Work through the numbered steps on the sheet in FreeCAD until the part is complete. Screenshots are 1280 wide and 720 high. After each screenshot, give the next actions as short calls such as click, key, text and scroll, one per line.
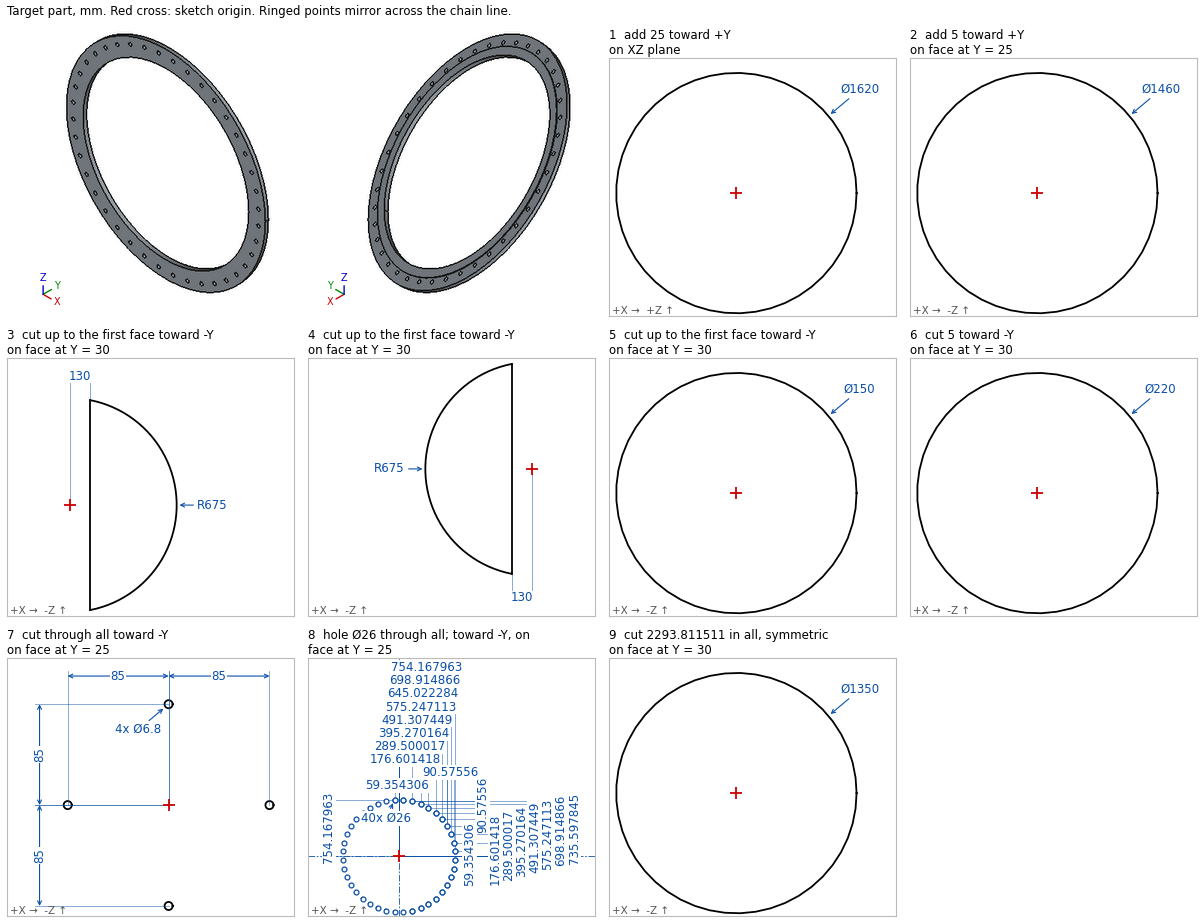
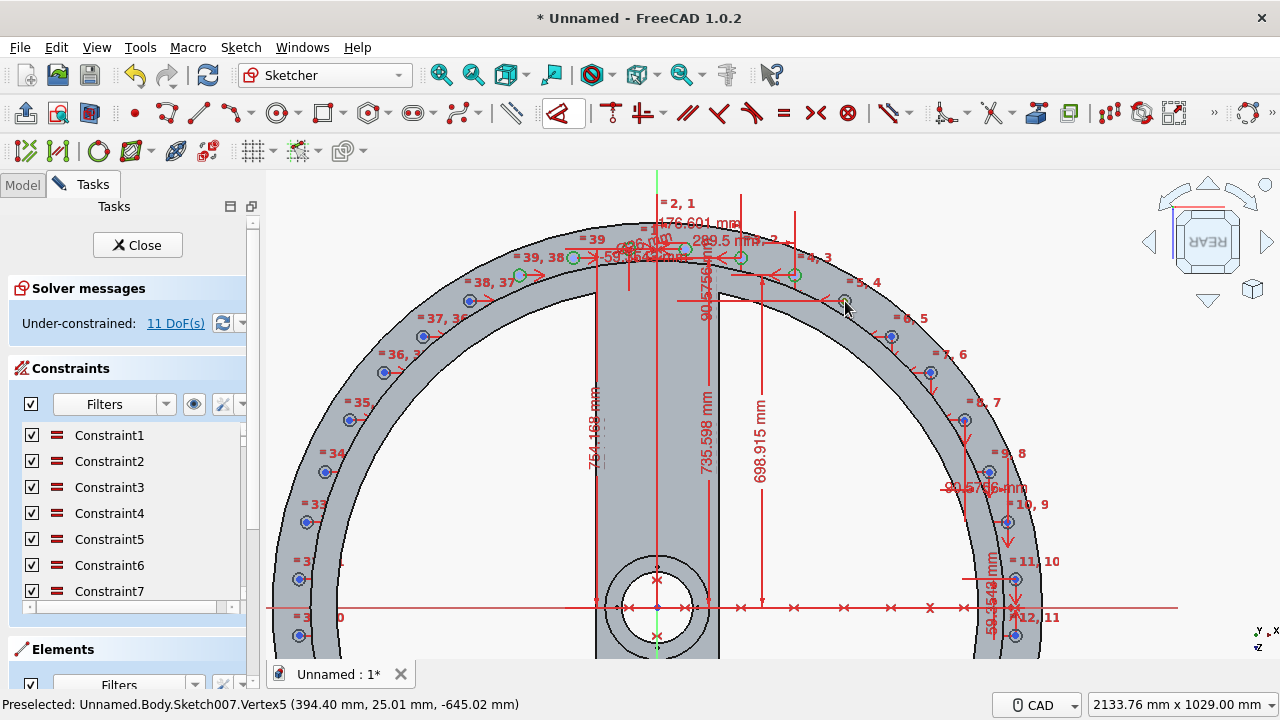
key(l)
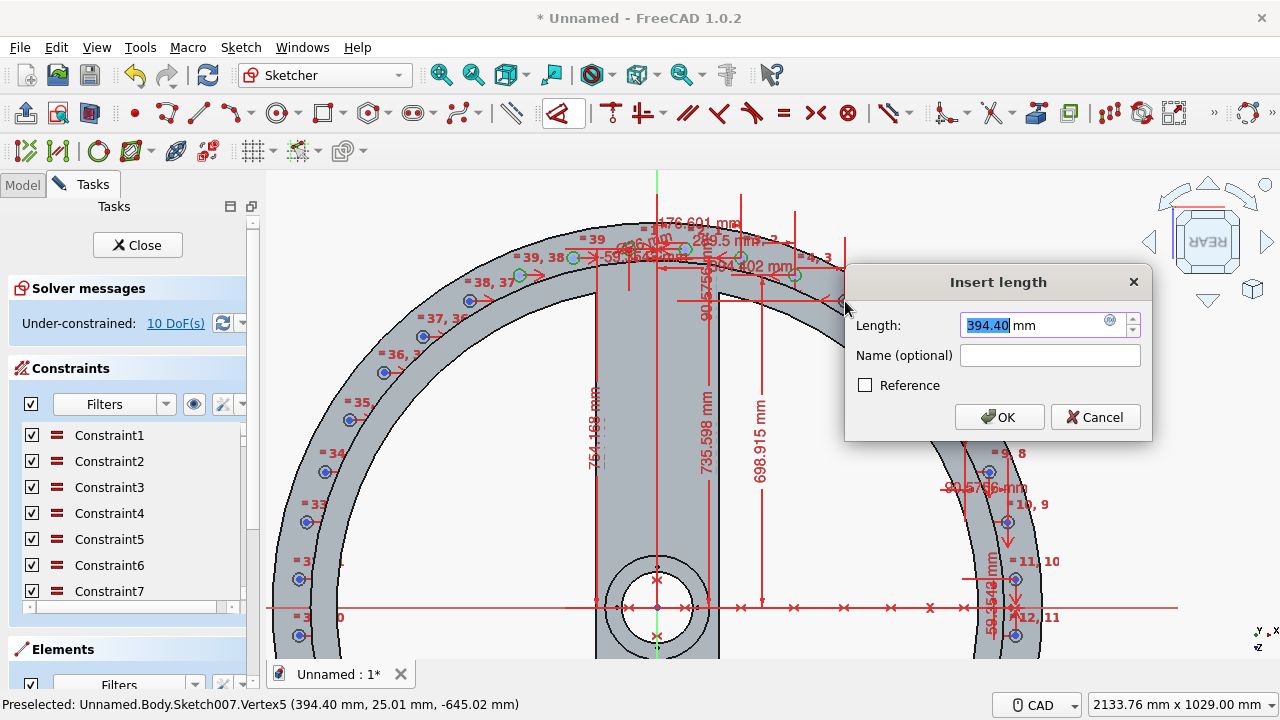
text(395.270164)
key(Return)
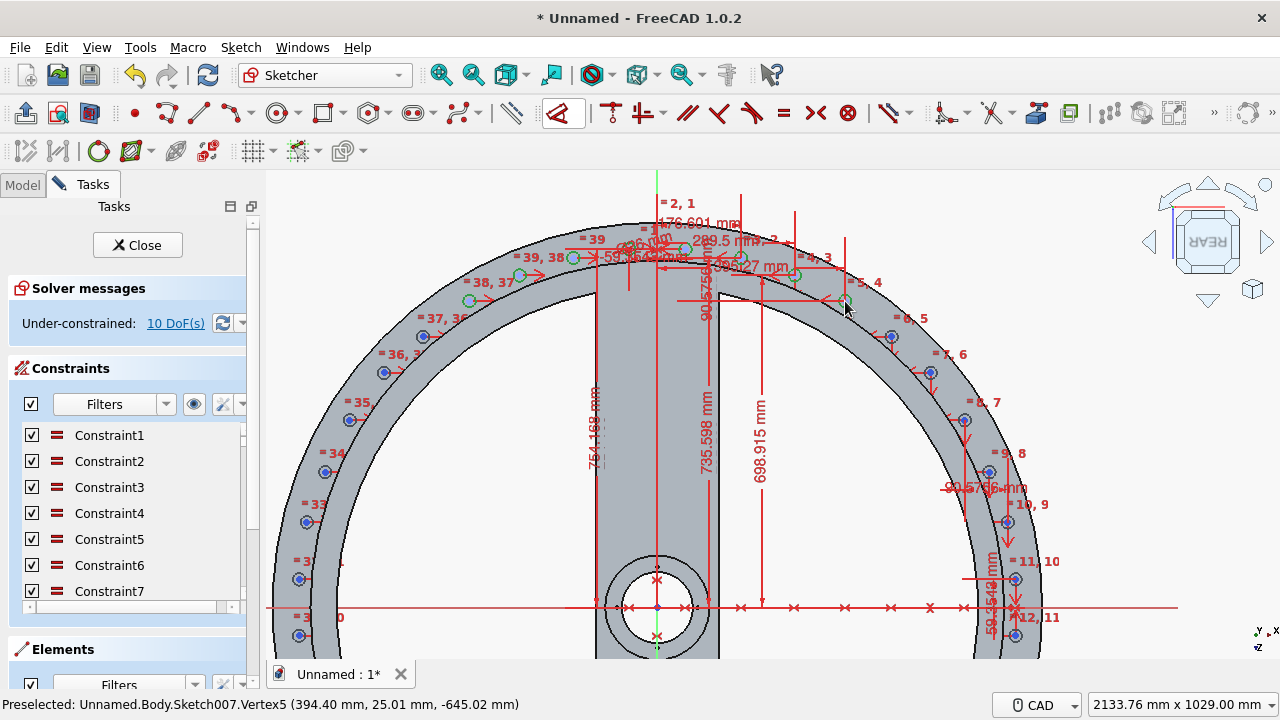
click(892, 337)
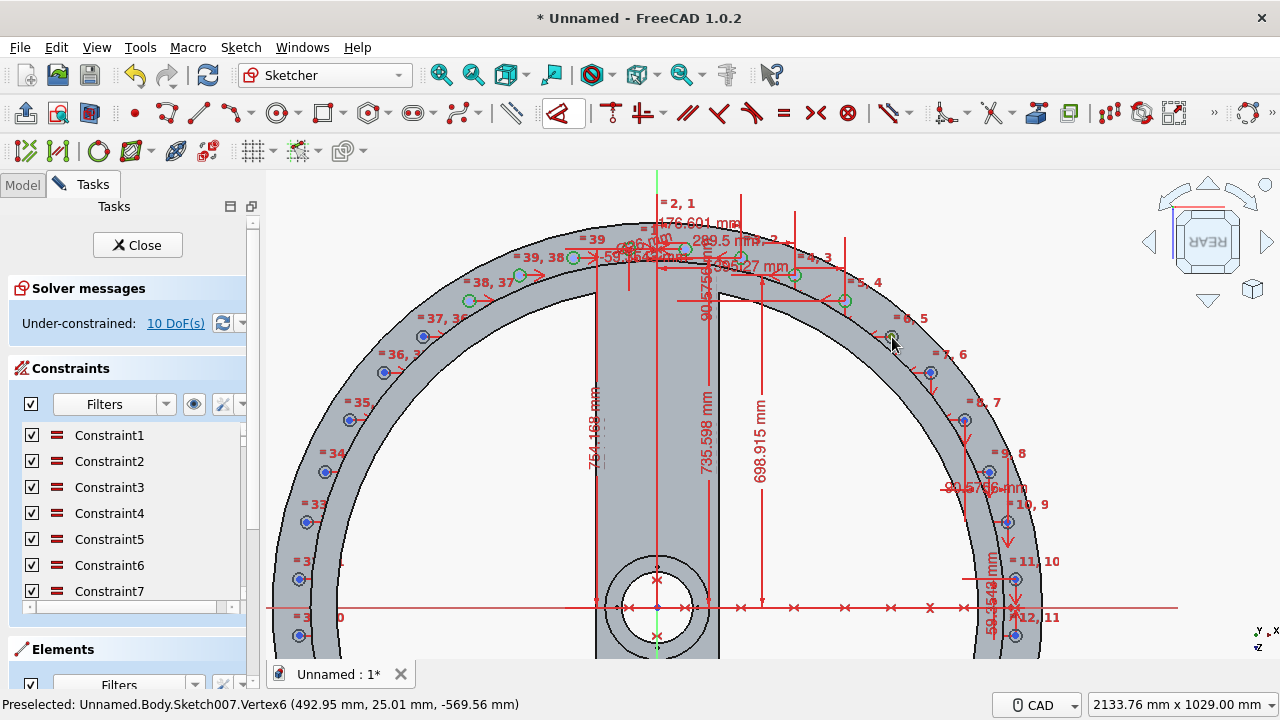
click(580, 114)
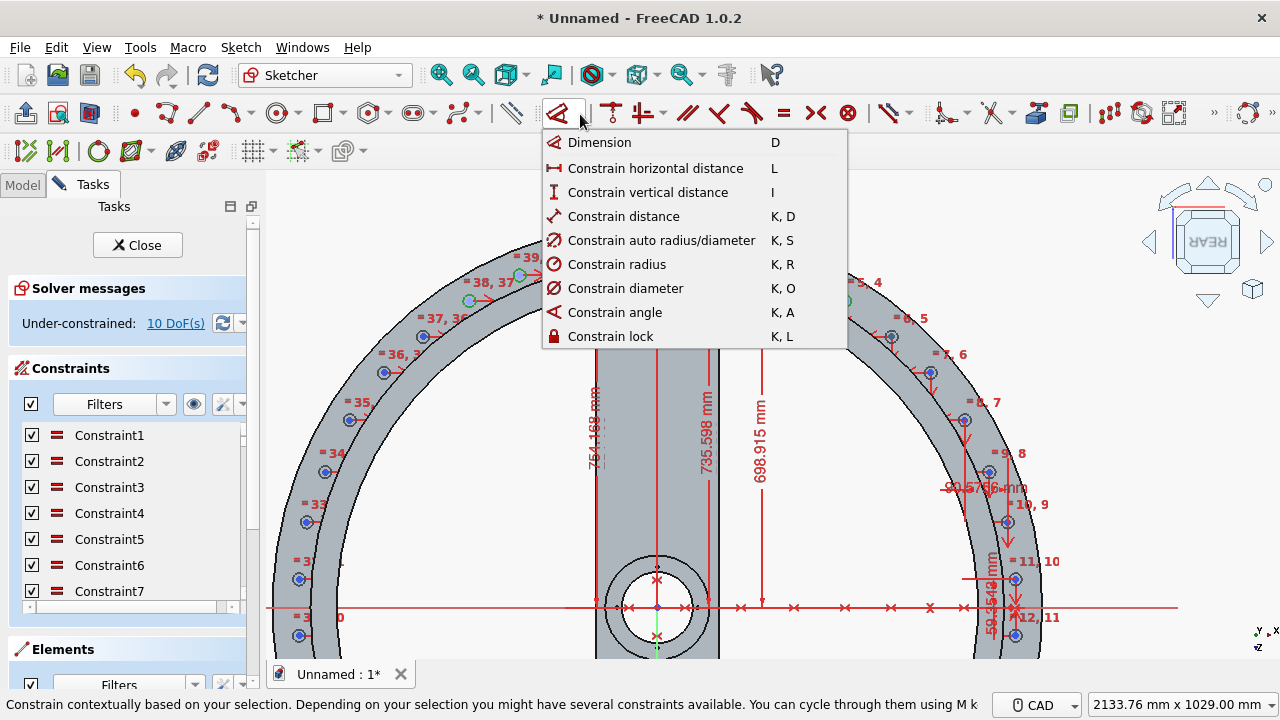
click(695, 168)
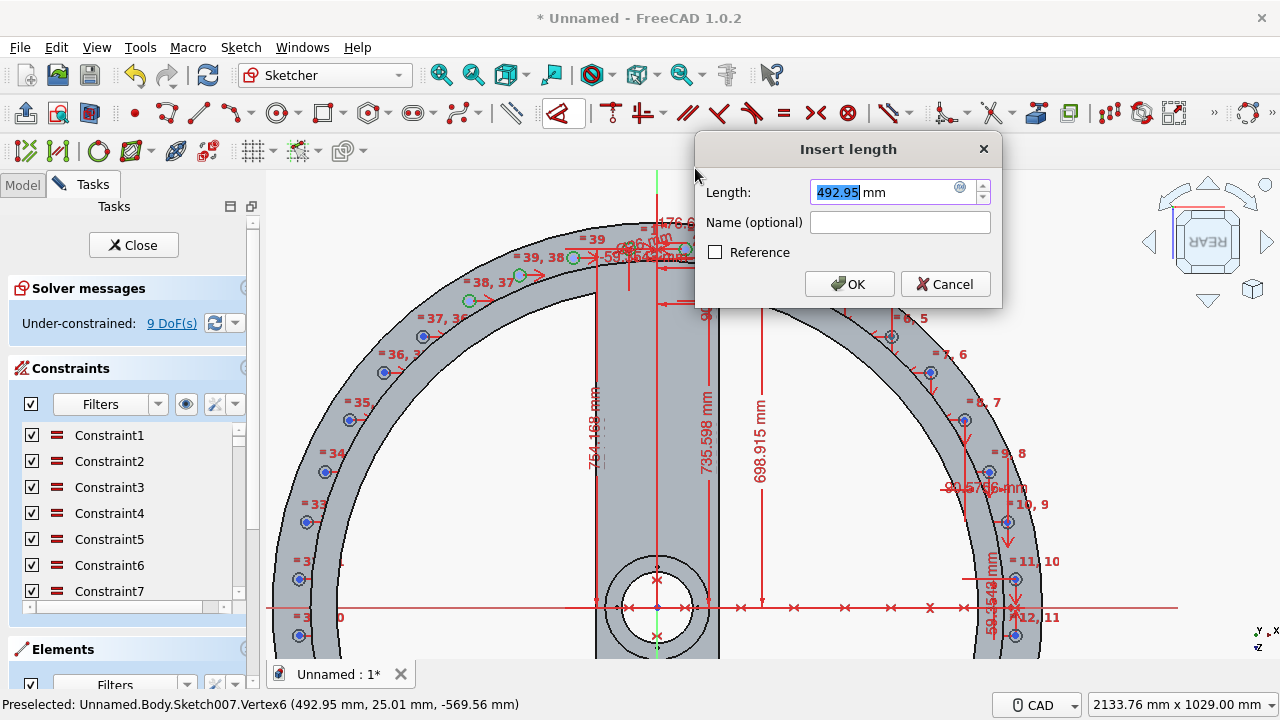
text(491.307449)
key(Return)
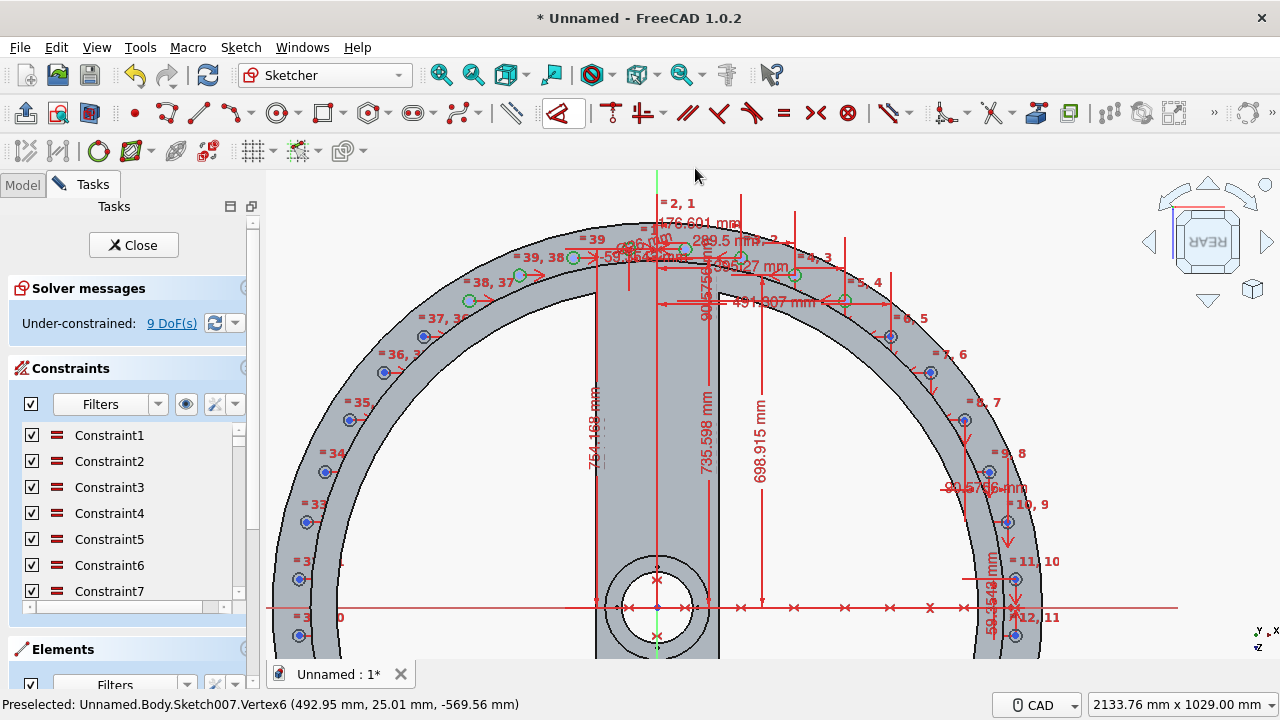
click(891, 337)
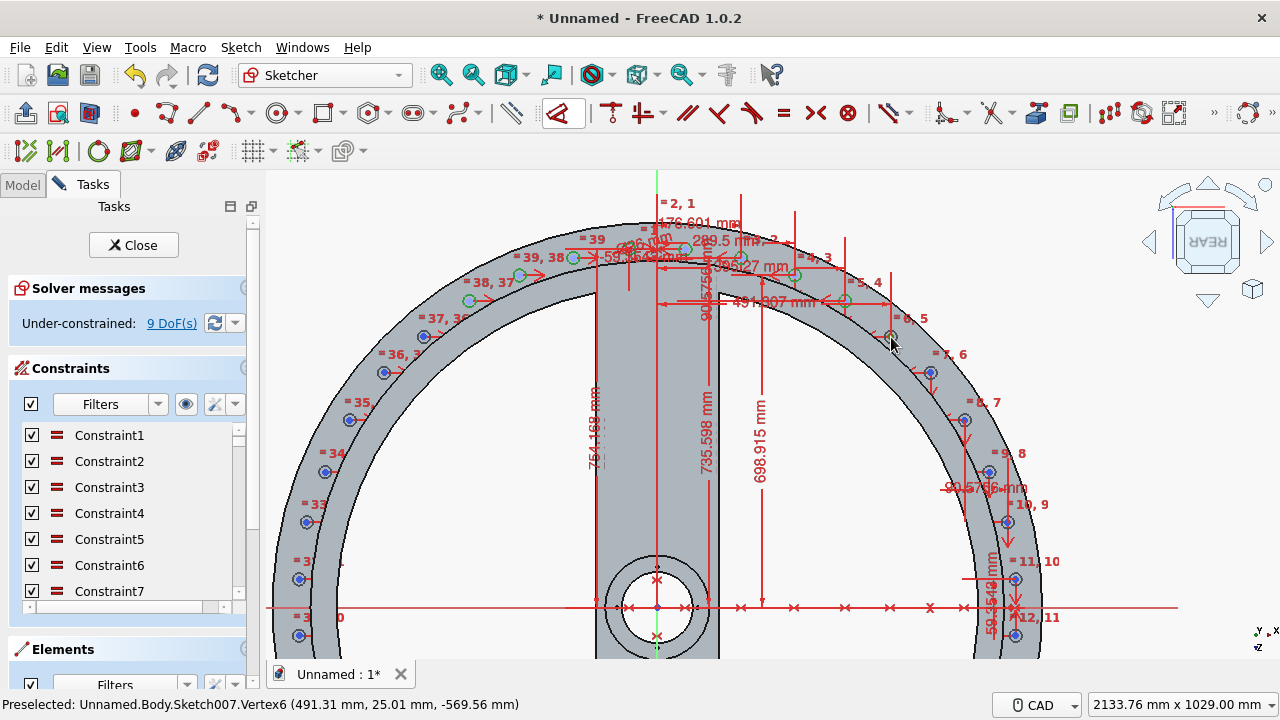
key(i)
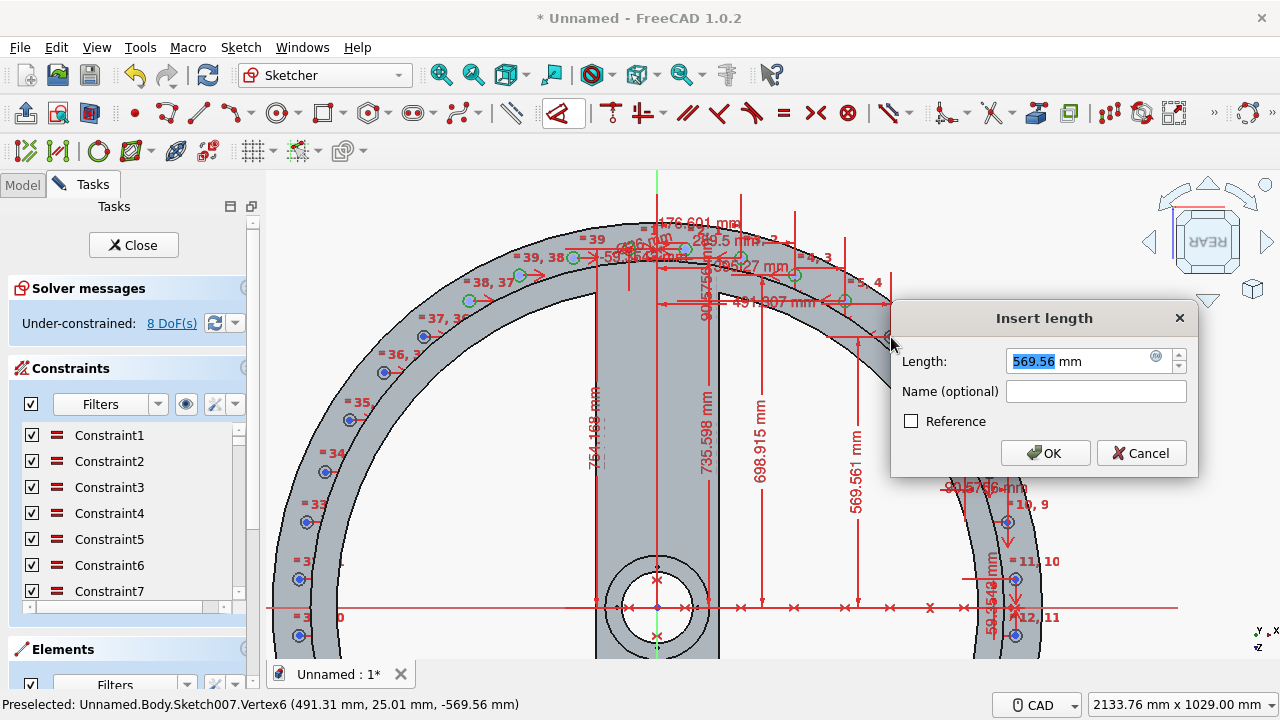
text(575.247113)
key(Return)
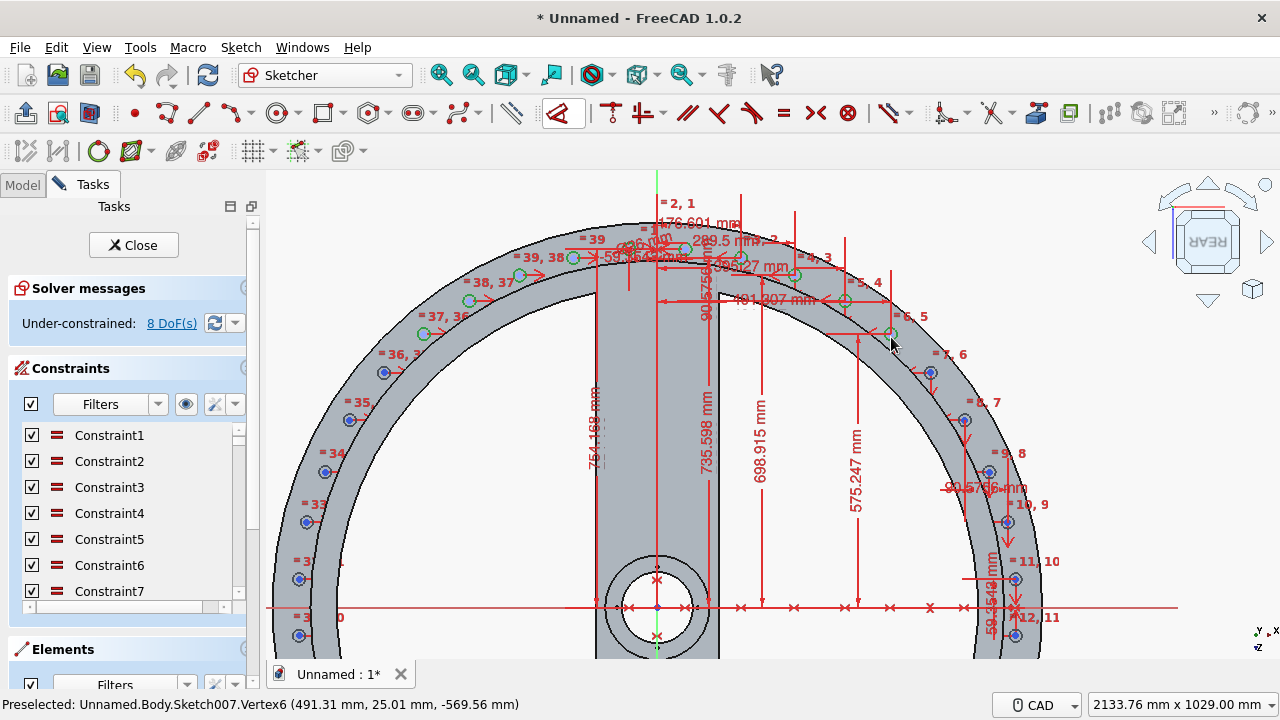
click(931, 373)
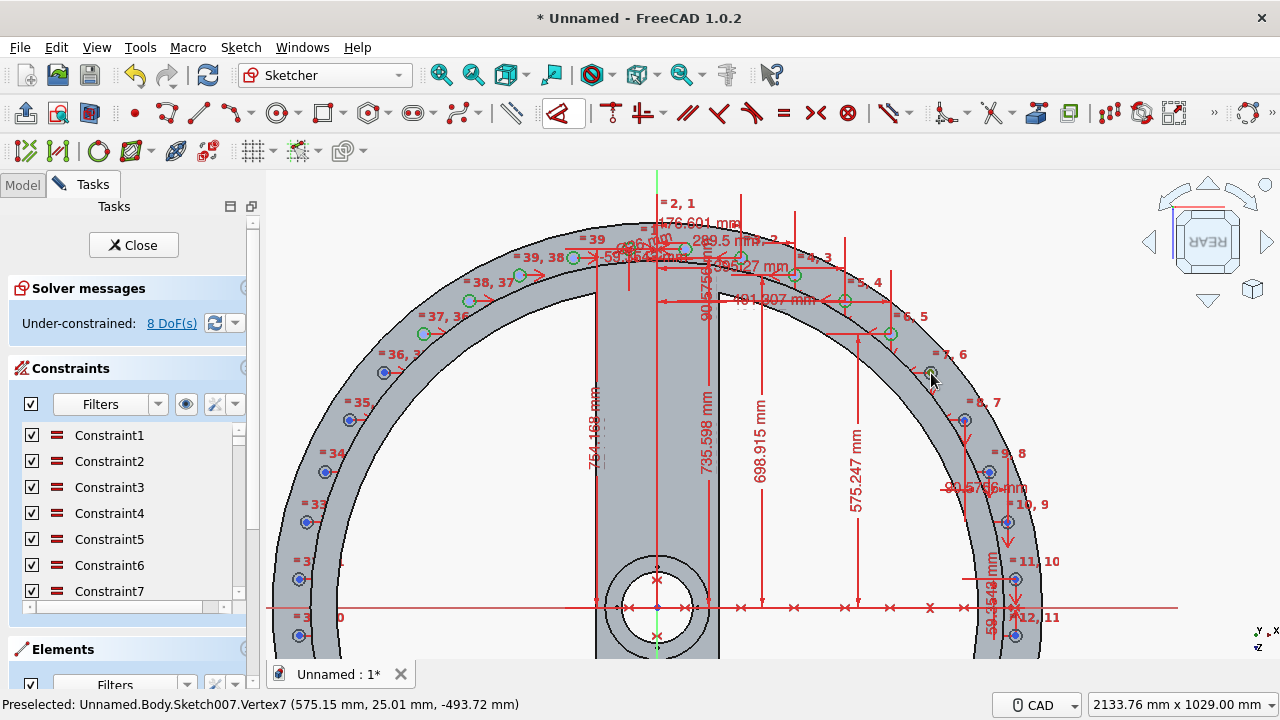
click(580, 114)